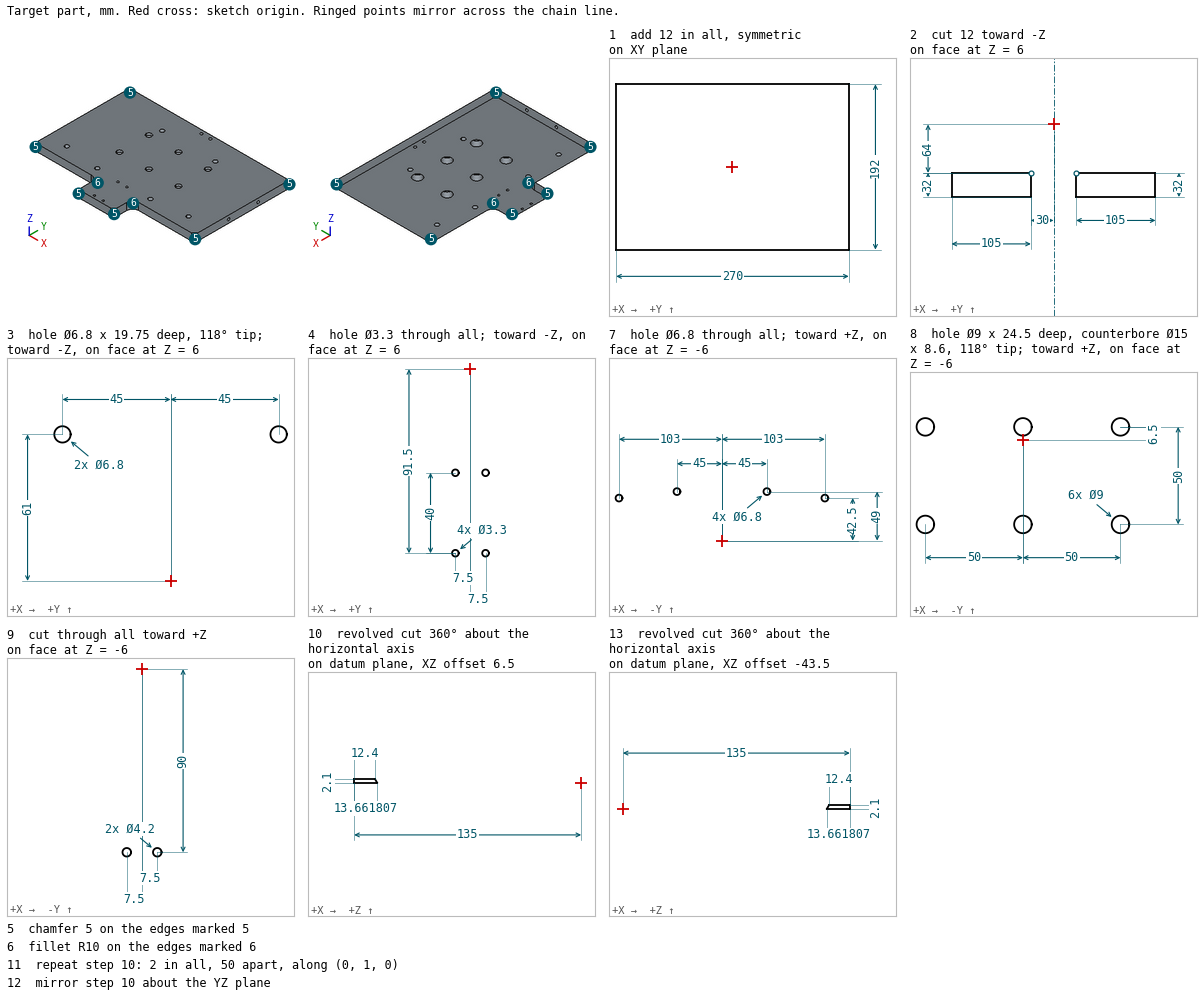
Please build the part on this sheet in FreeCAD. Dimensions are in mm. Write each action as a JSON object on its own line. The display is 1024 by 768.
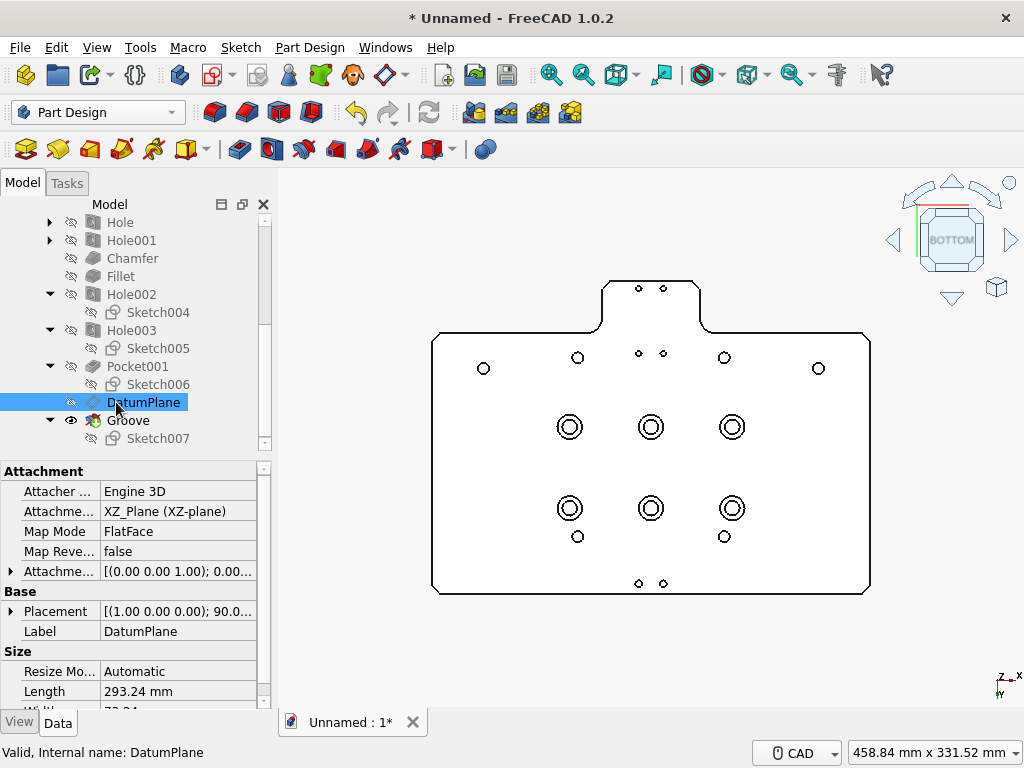
{"action": "left_click", "coordinate": [116, 420]}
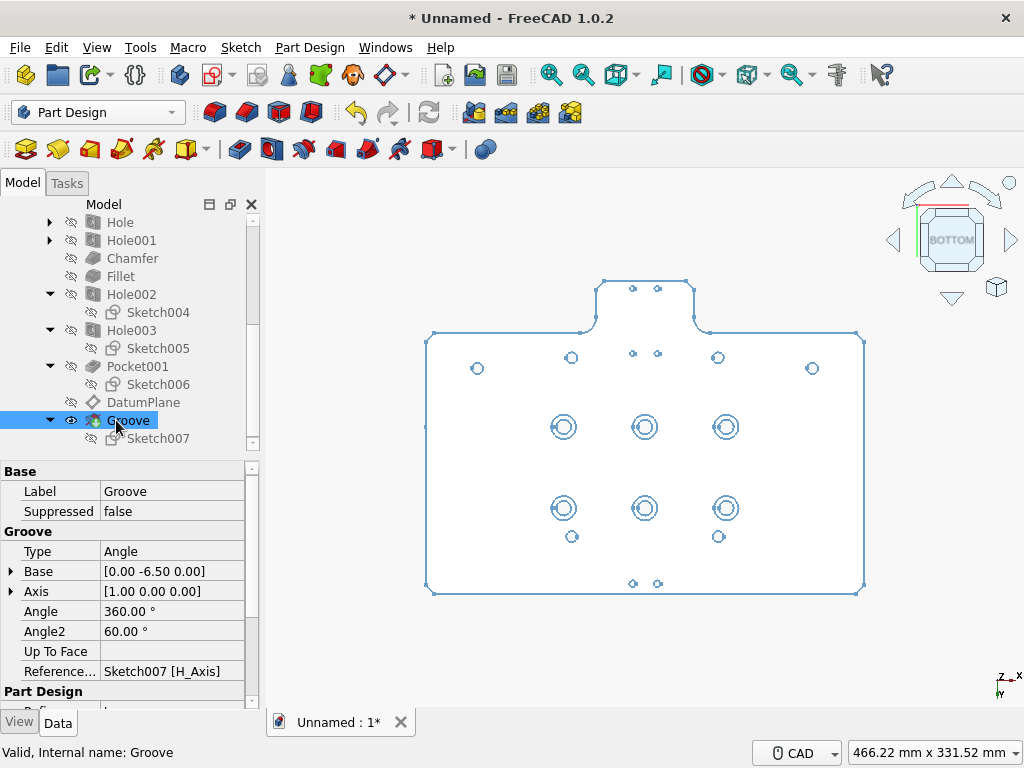
{"action": "left_click", "coordinate": [506, 112]}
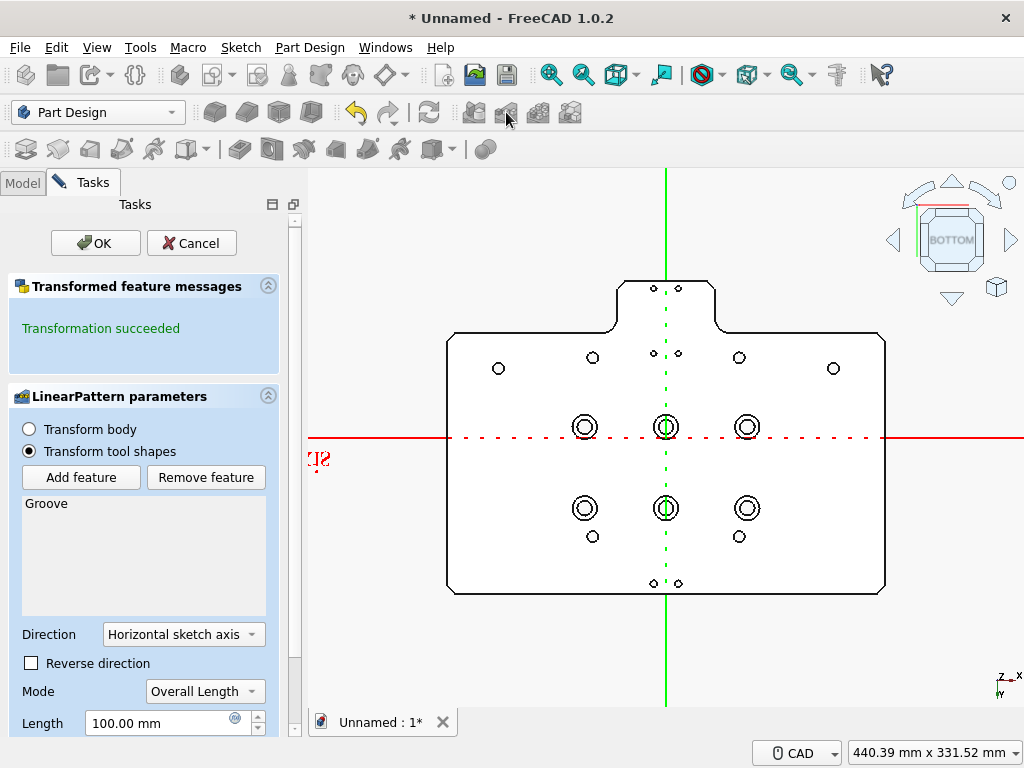
{"action": "left_click", "coordinate": [184, 634]}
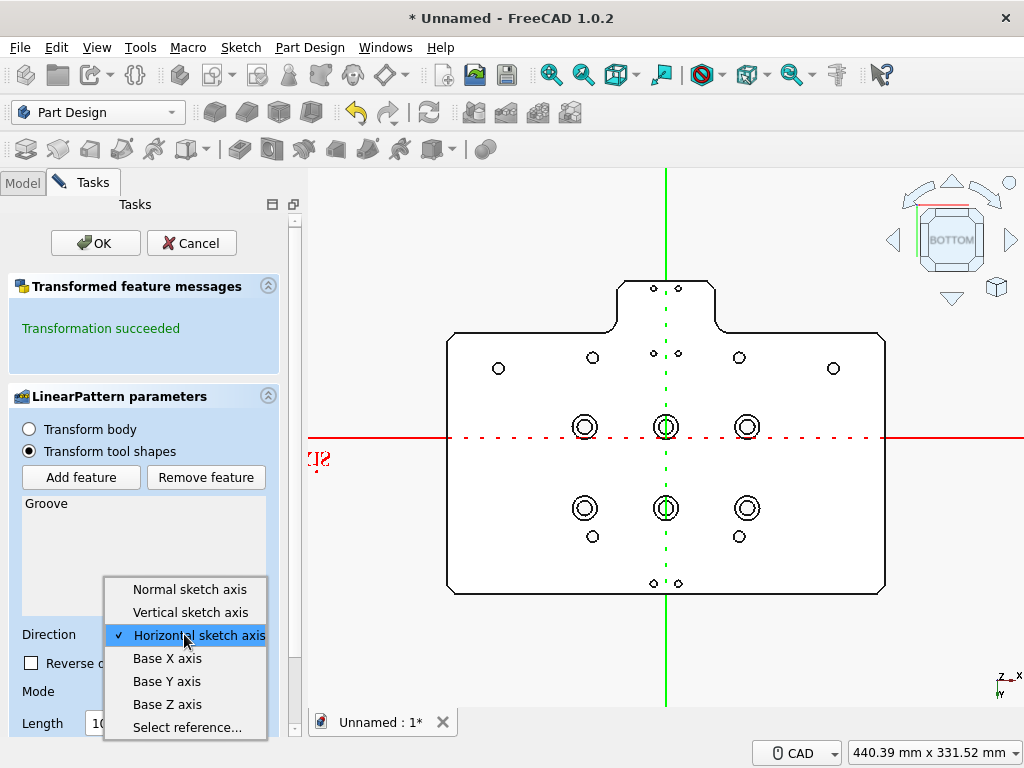
{"action": "left_click", "coordinate": [184, 682]}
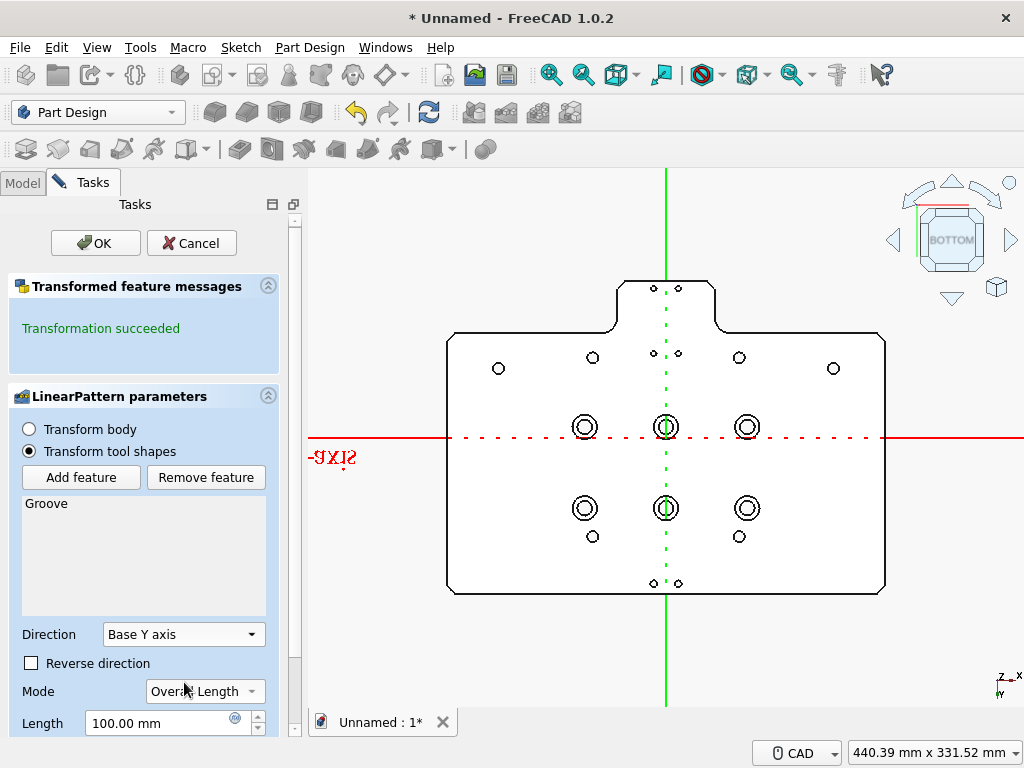
{"action": "left_click", "coordinate": [206, 692]}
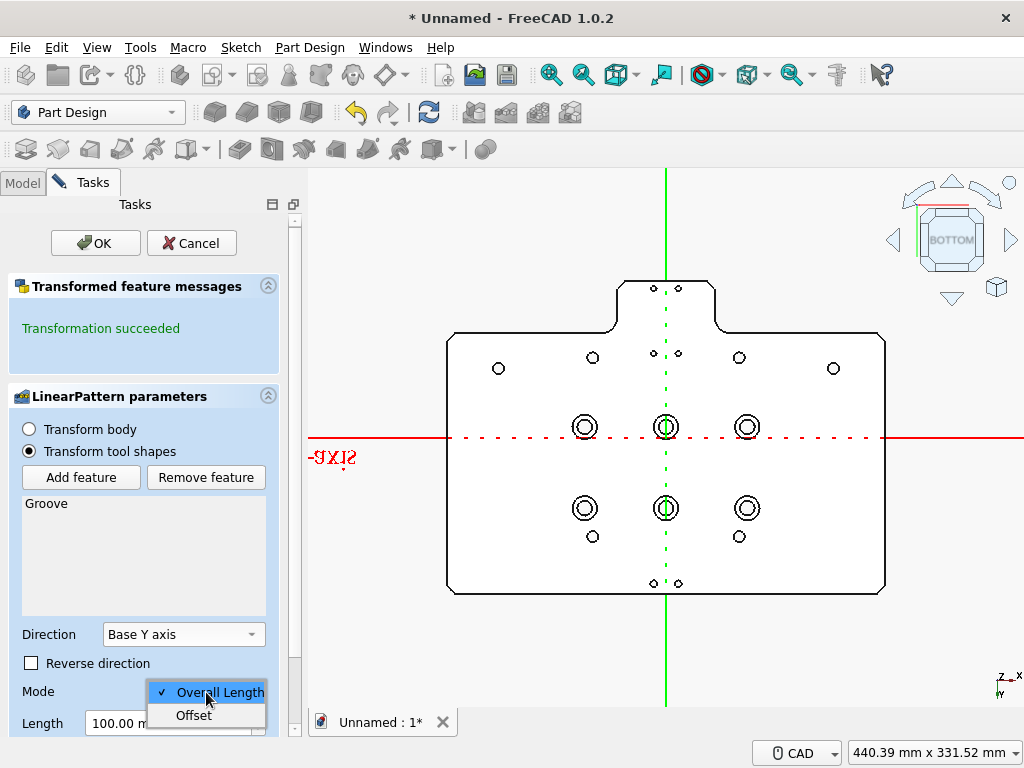
{"action": "left_click", "coordinate": [206, 716]}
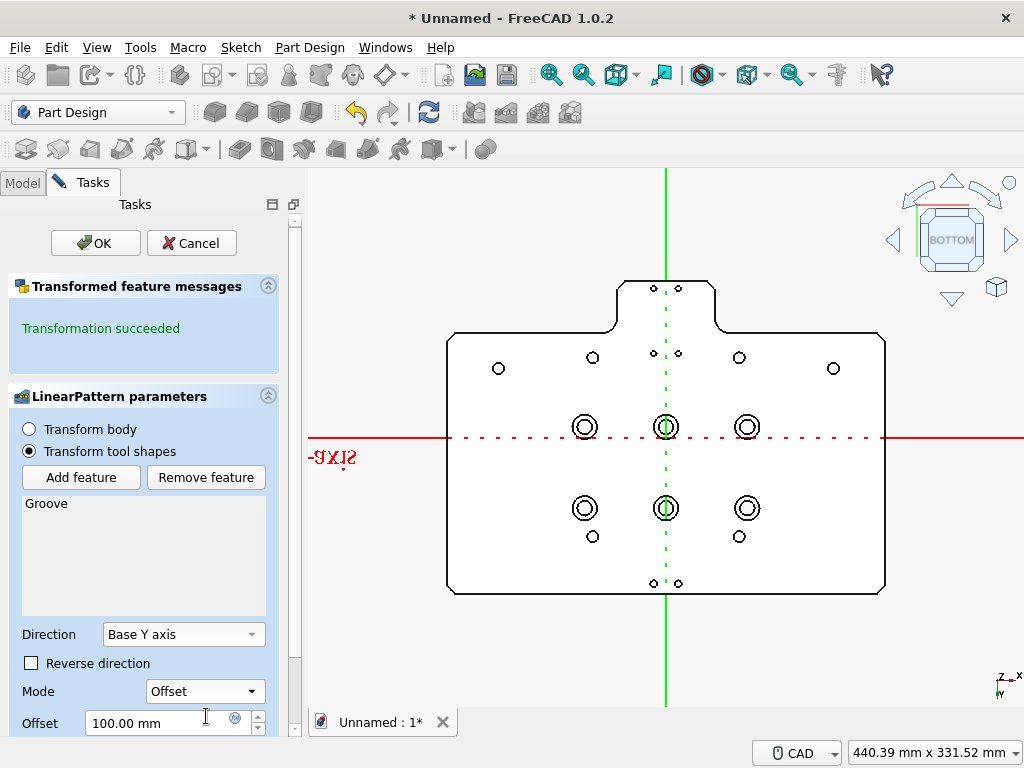
{"action": "triple_click", "coordinate": [168, 723]}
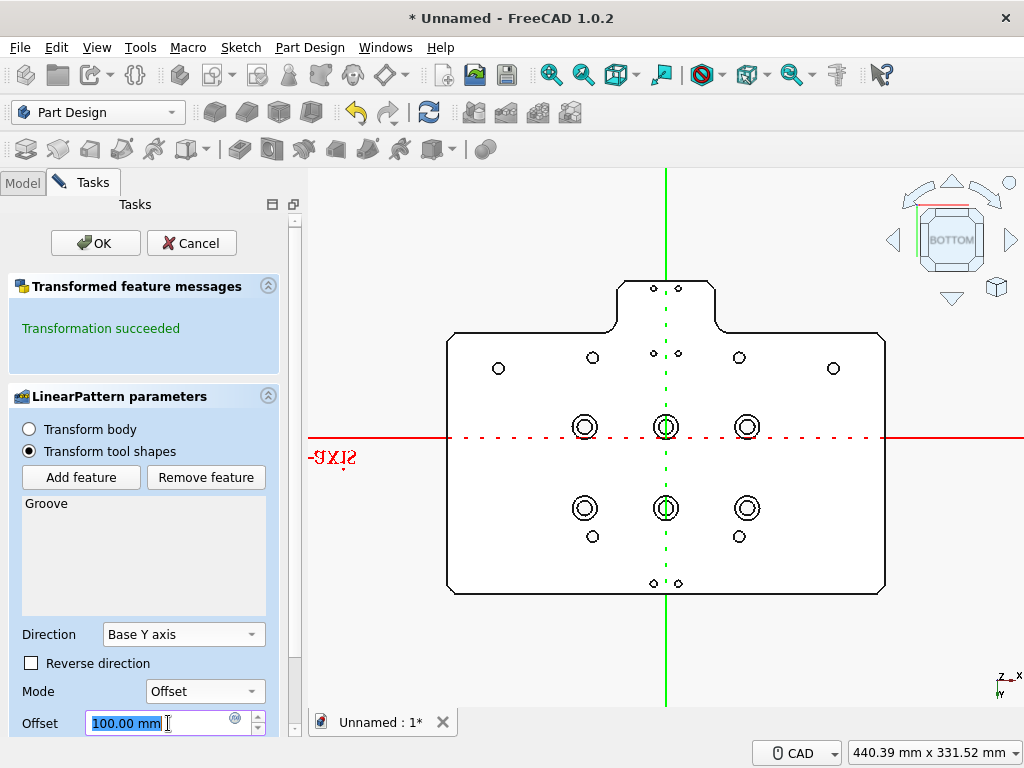
{"action": "type", "text": "50"}
{"action": "key", "text": "Tab"}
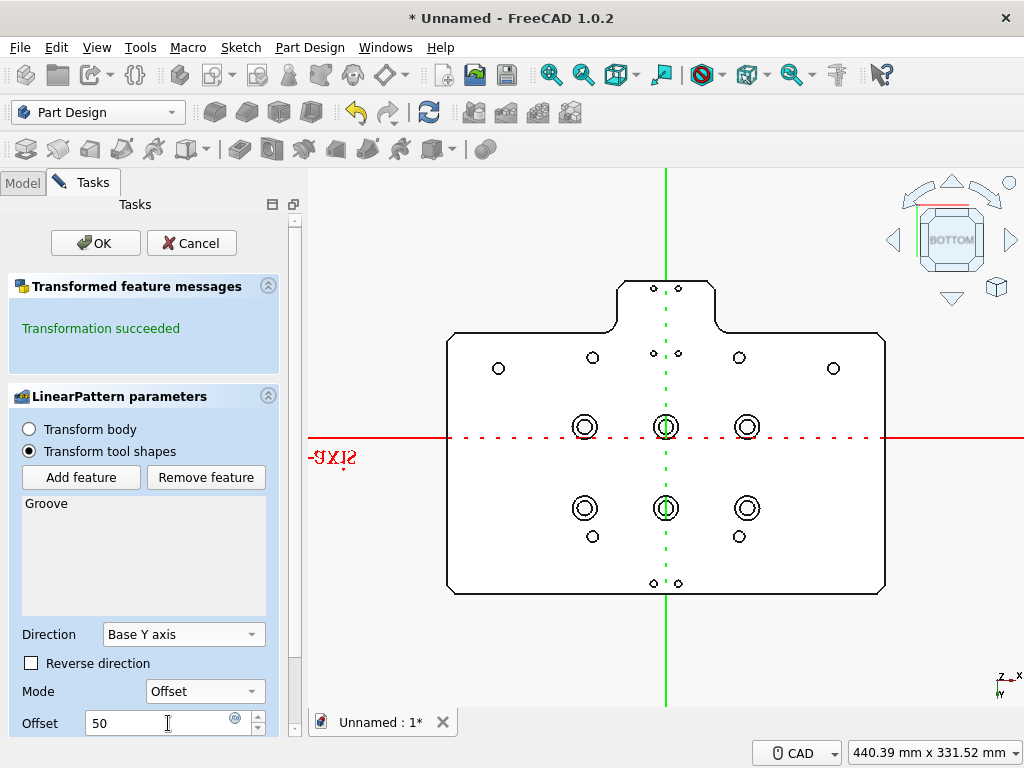
{"action": "scroll", "coordinate": [295, 475], "scroll_direction": "down", "scroll_amount": 2}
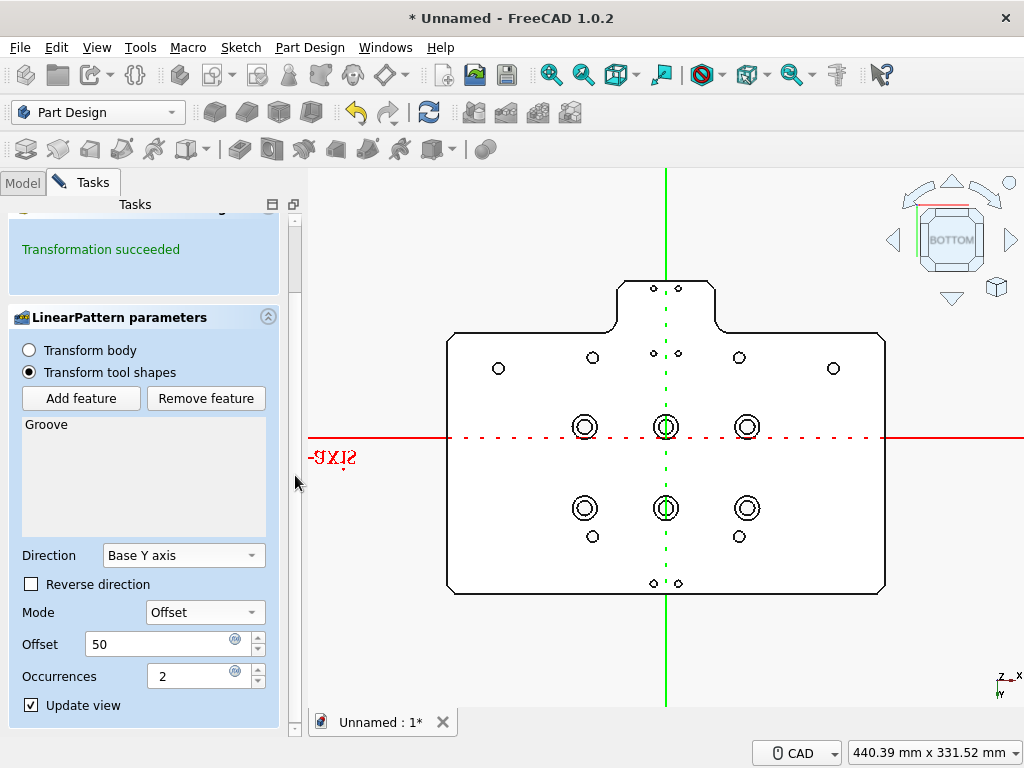
{"action": "triple_click", "coordinate": [198, 676]}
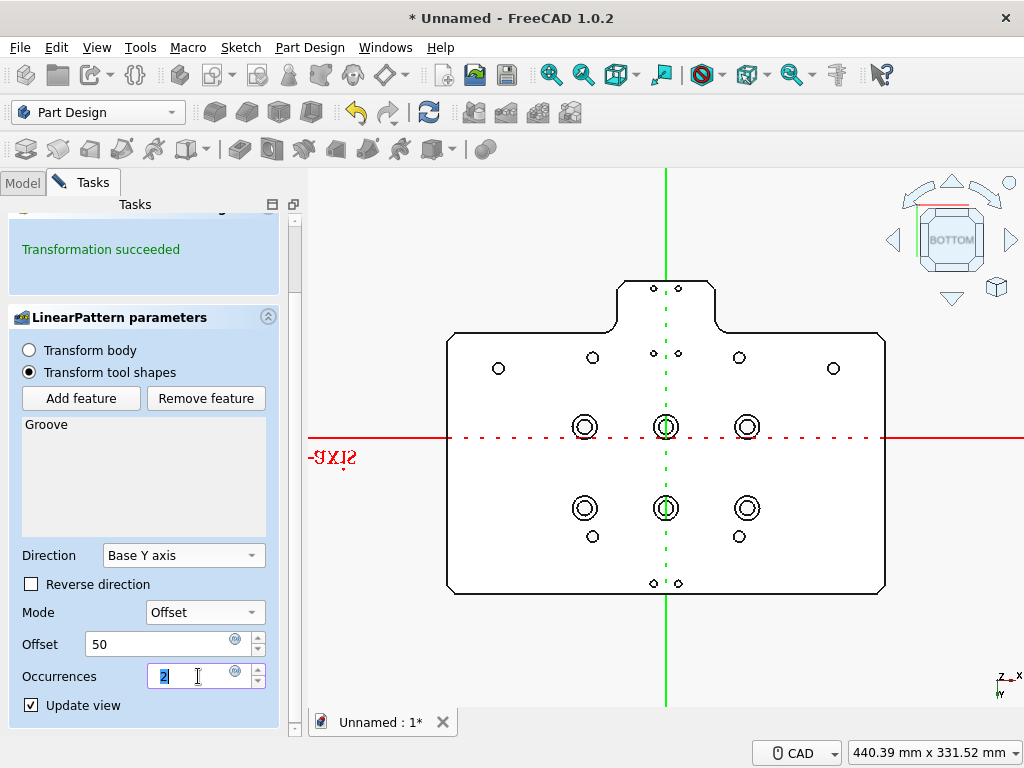
{"action": "type", "text": "2"}
{"action": "key", "text": "Tab"}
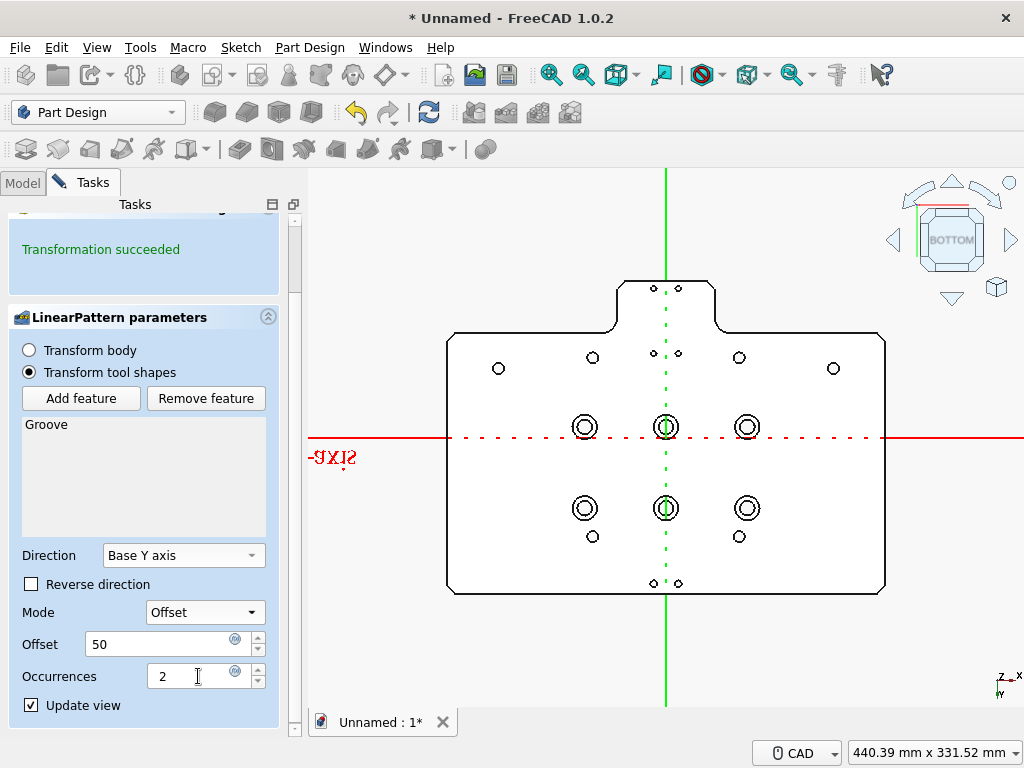
{"action": "scroll", "coordinate": [295, 475], "scroll_direction": "up", "scroll_amount": 3}